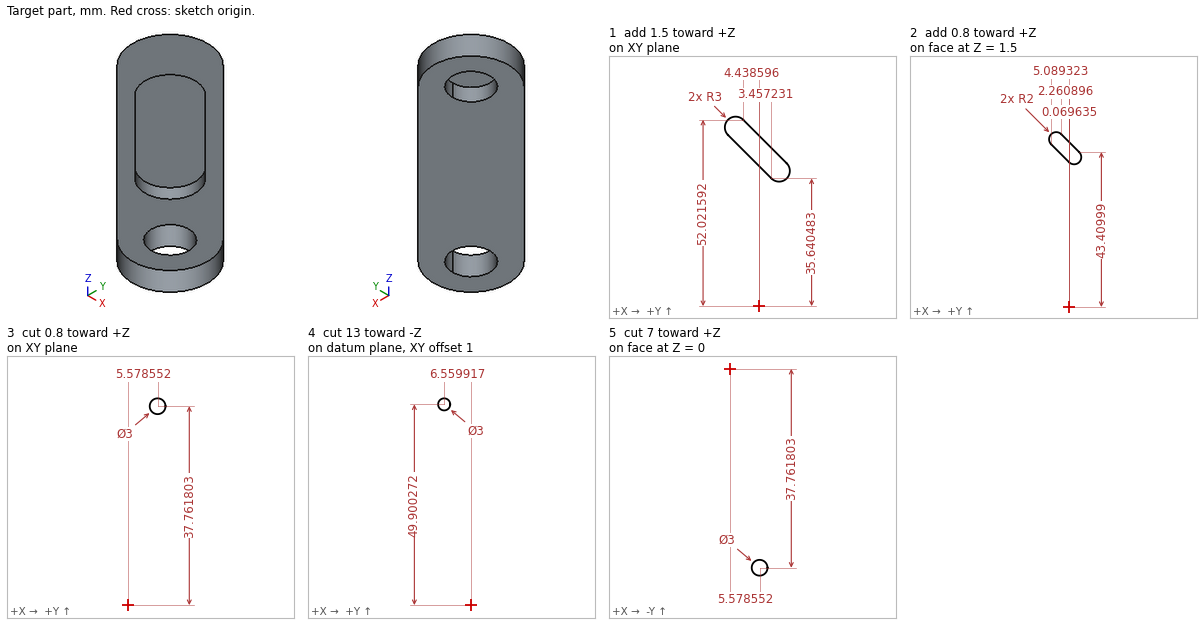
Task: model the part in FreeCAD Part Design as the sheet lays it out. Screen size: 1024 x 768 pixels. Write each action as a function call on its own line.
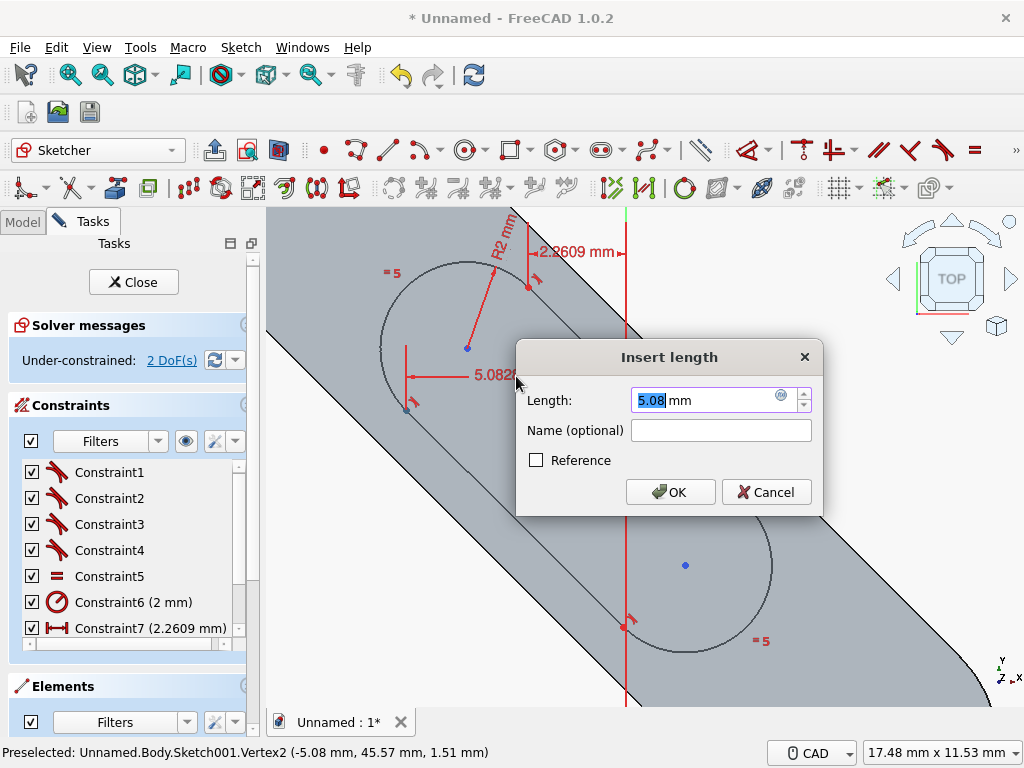
text(5.089323)
key(Return)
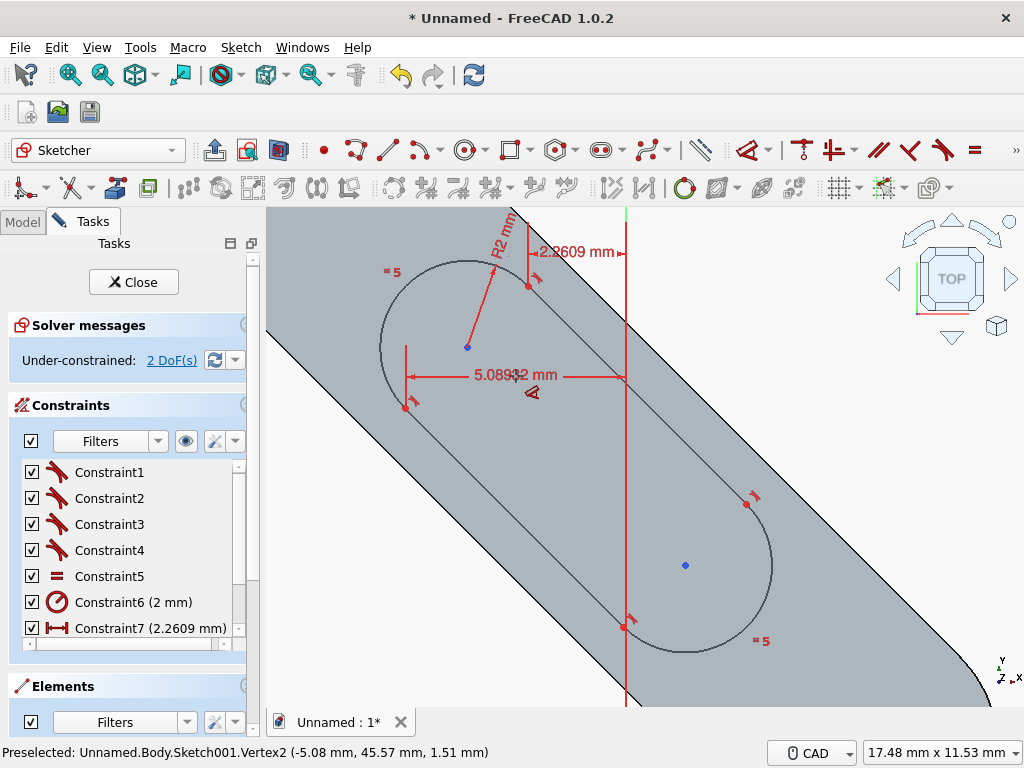
scroll(624, 627, up, 13)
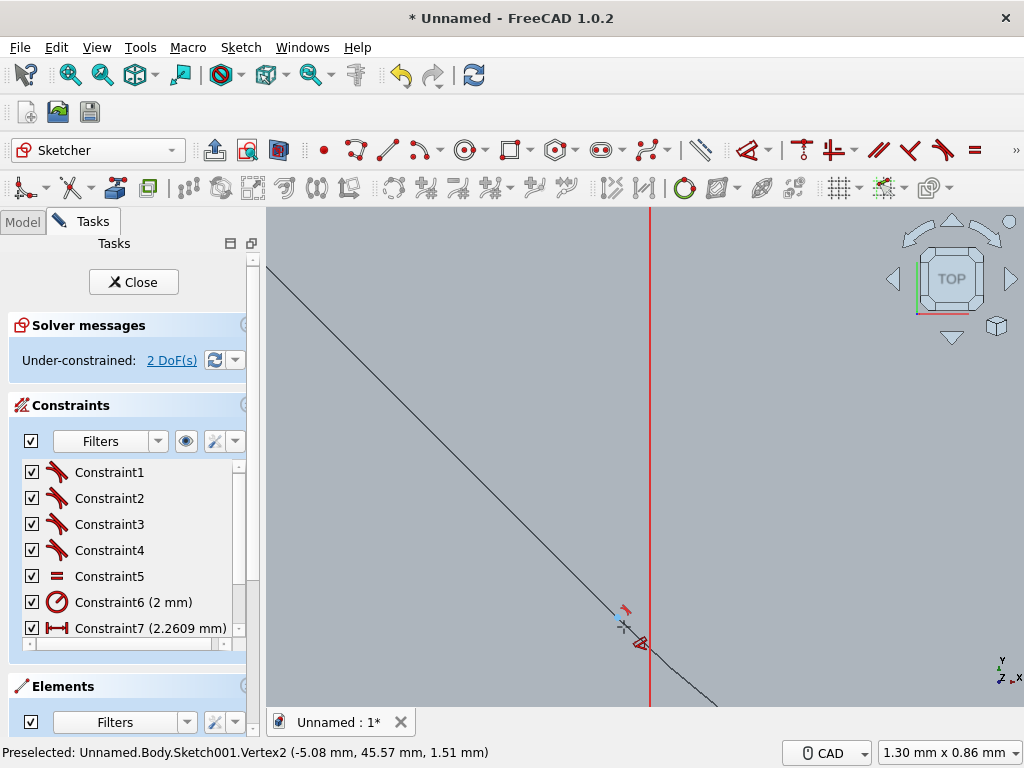
click(618, 618)
click(634, 584)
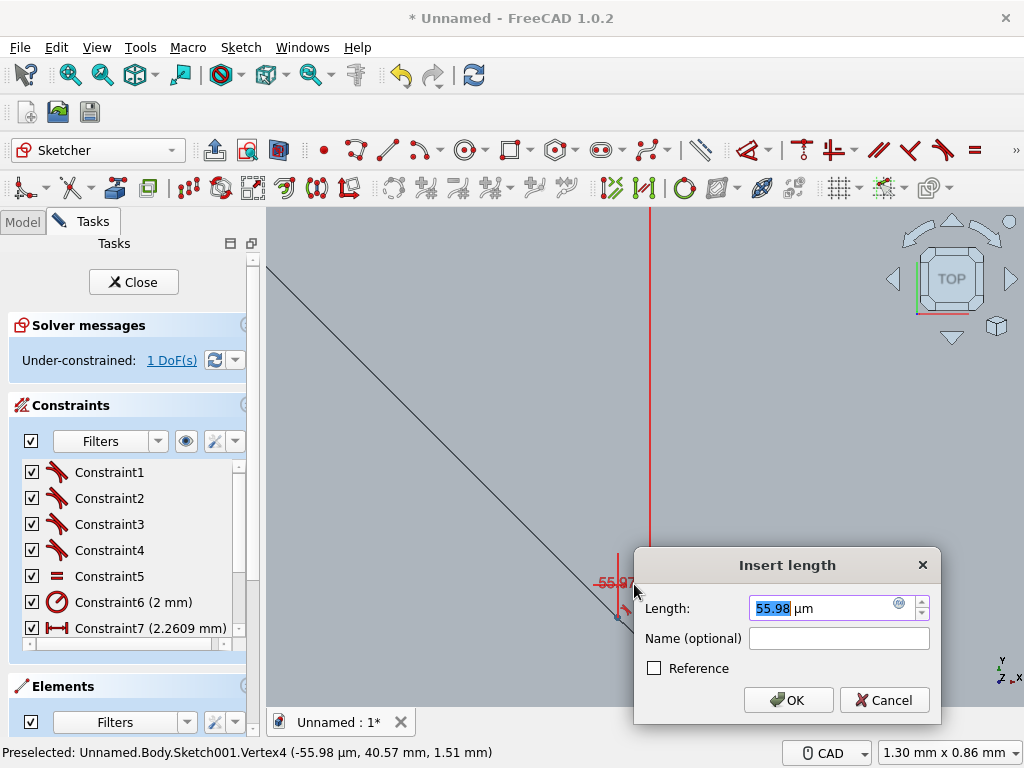
key(ctrl+a)
text(0.069635 mm)
key(Return)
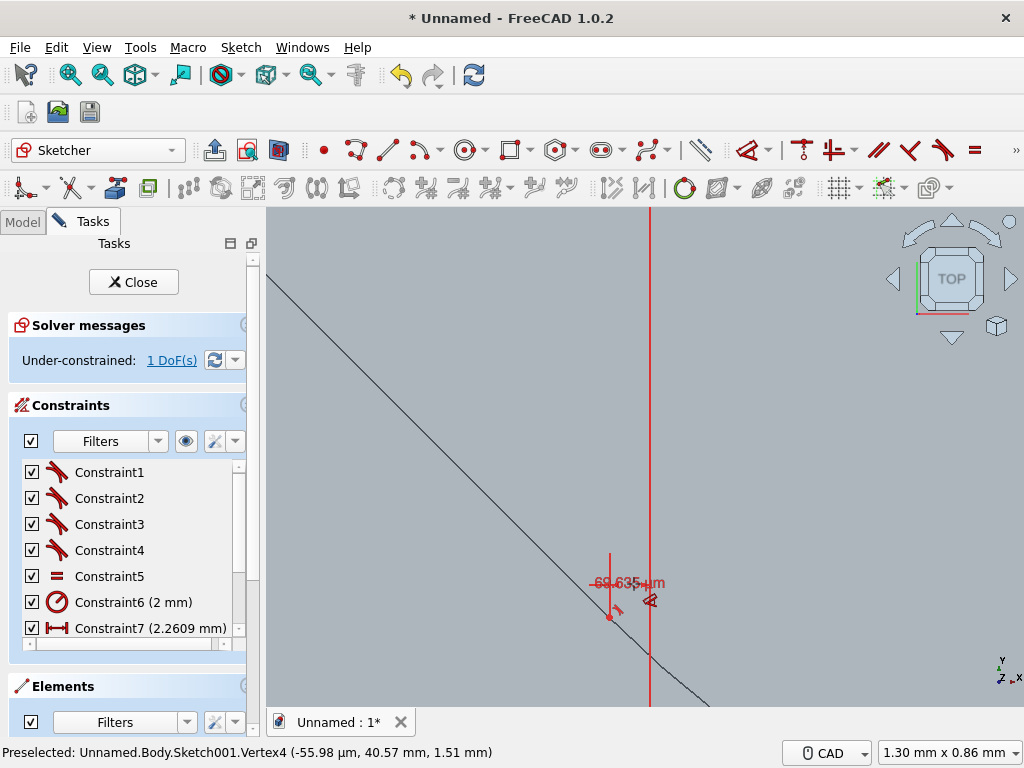
scroll(625, 628, down, 13)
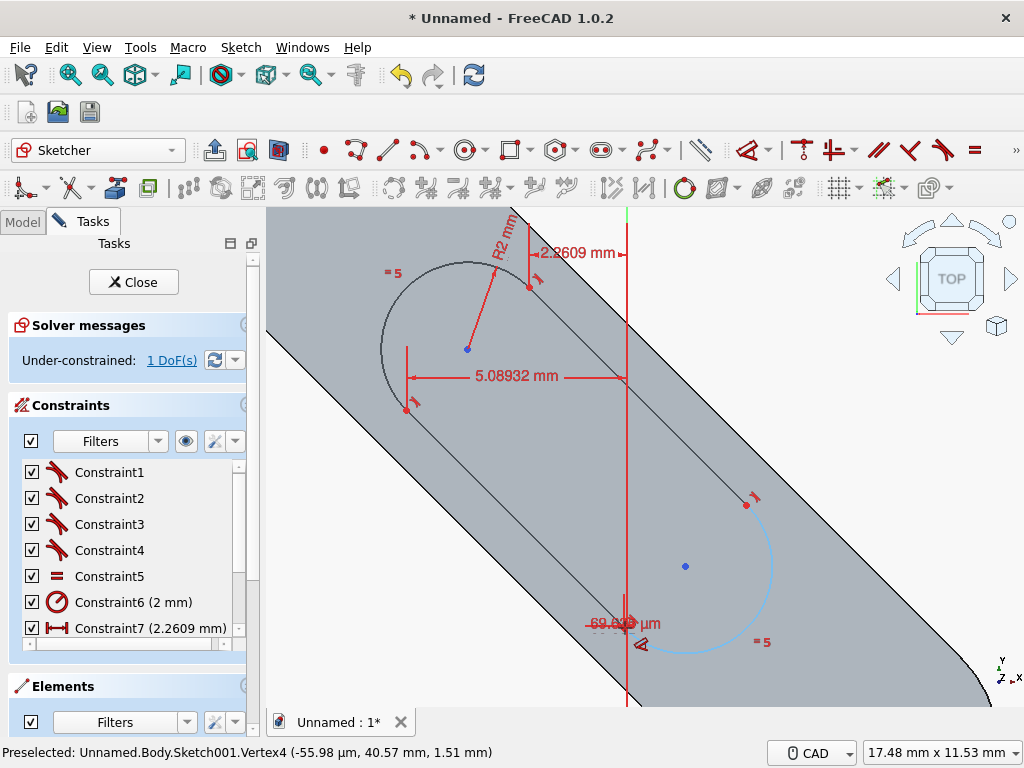
click(747, 505)
click(781, 632)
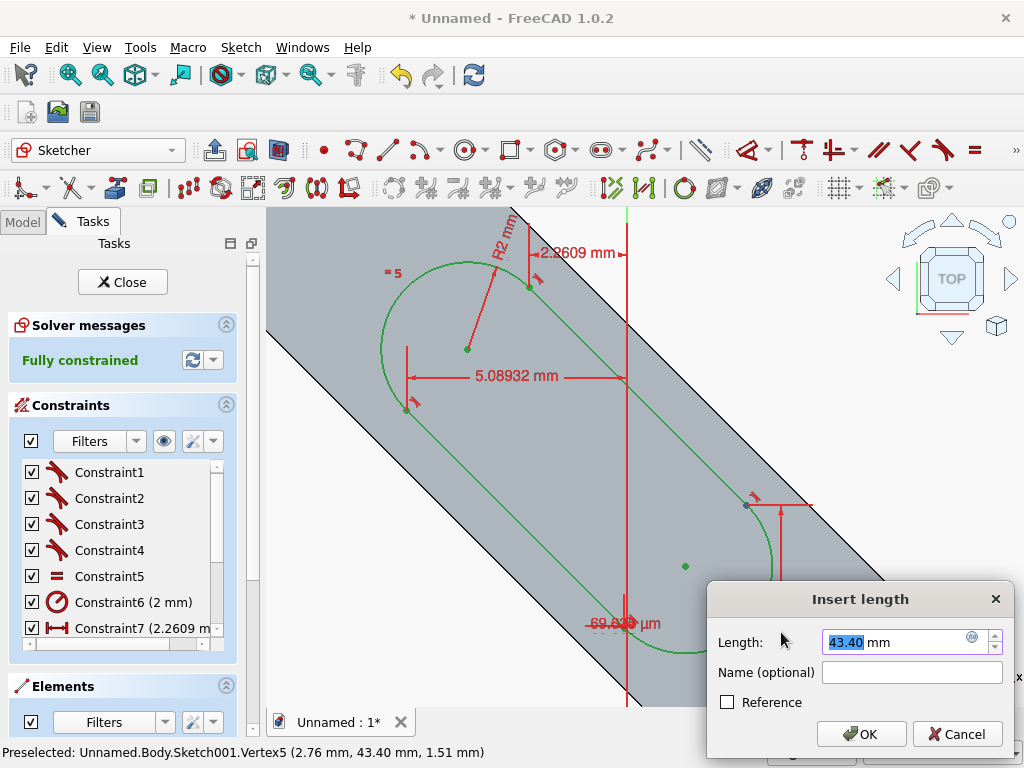
text(43.40999)
key(Return)
key(Escape)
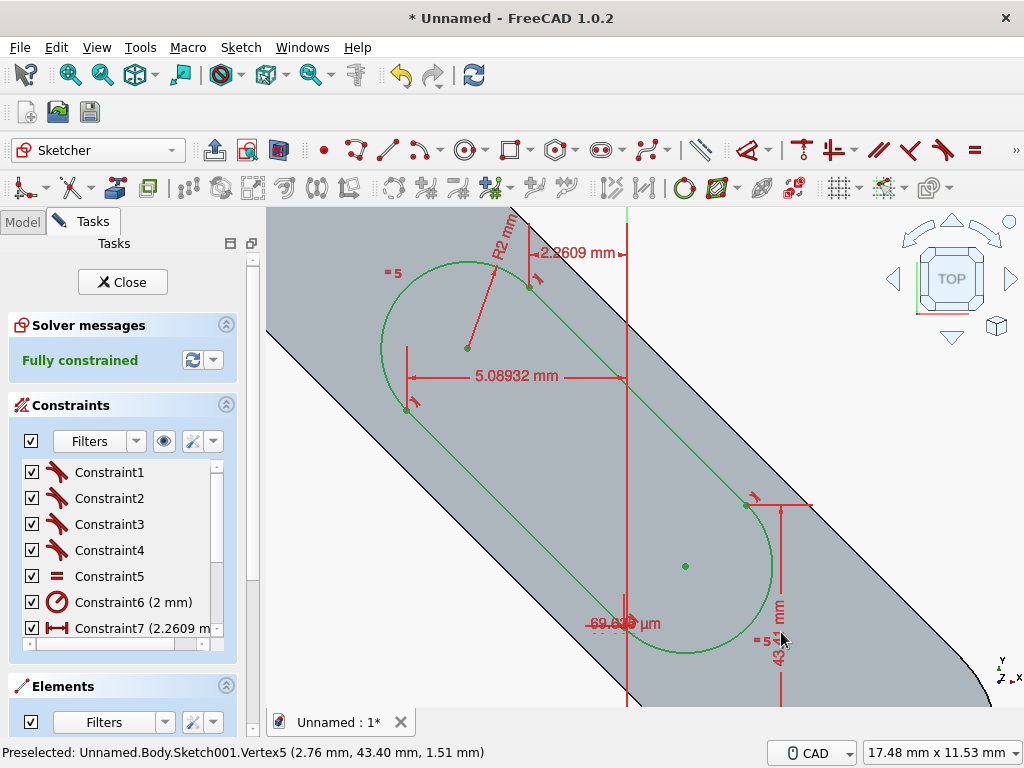
click(123, 282)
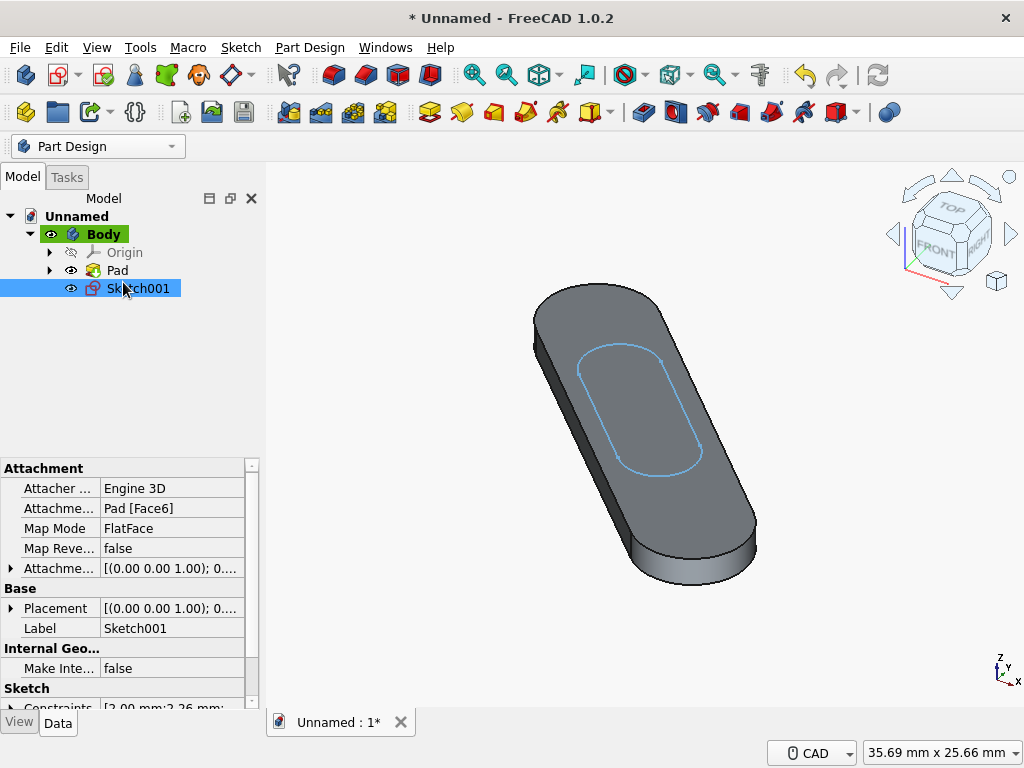
click(430, 112)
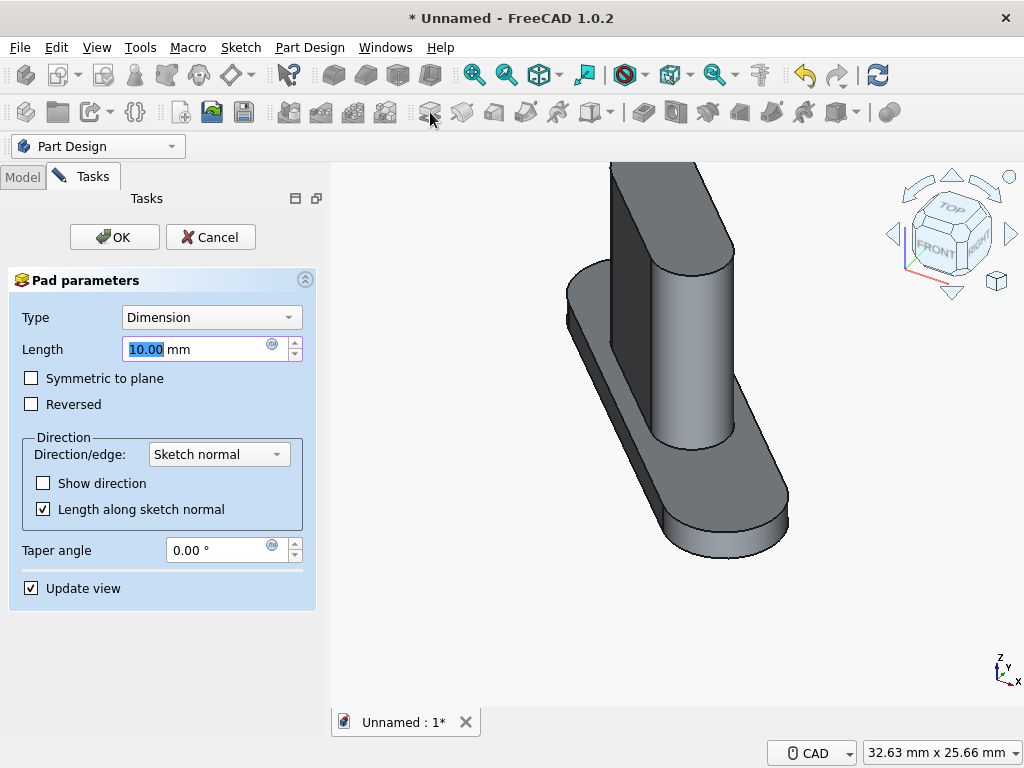
text(0.8)
key(Tab)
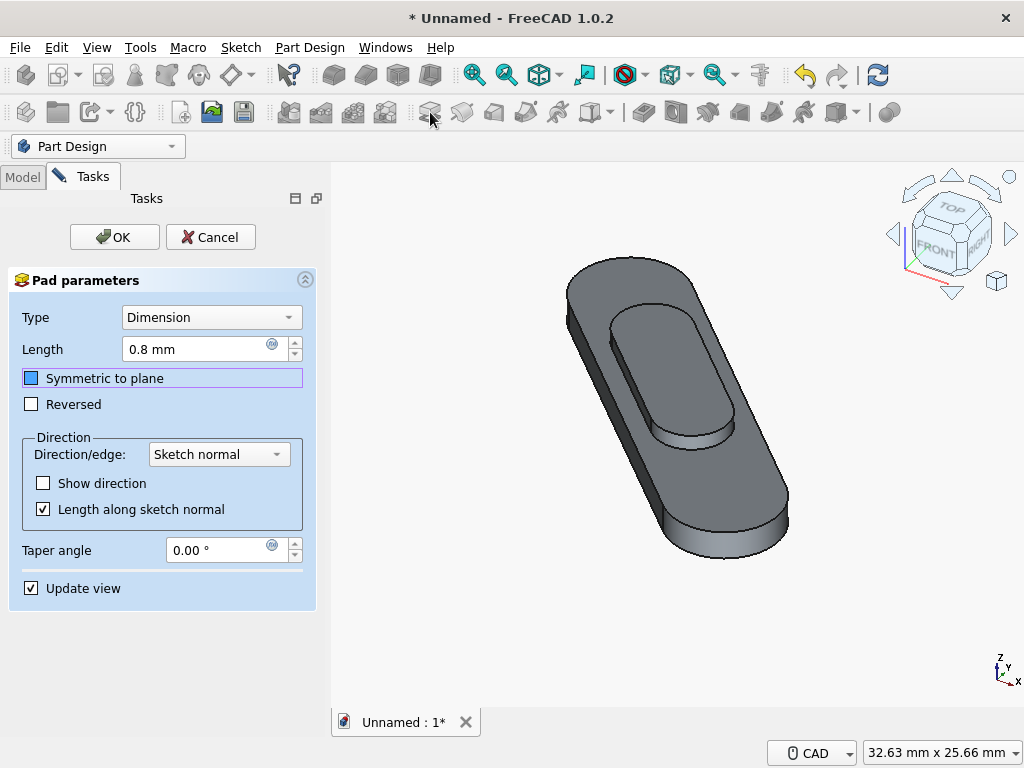
click(115, 237)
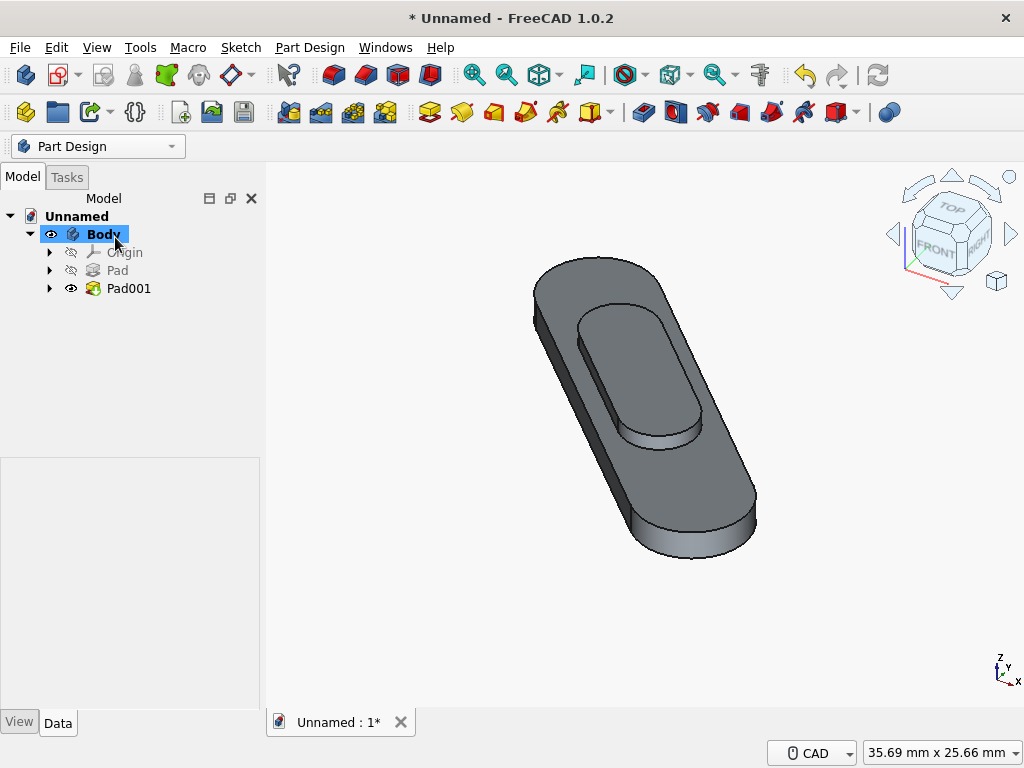
click(58, 76)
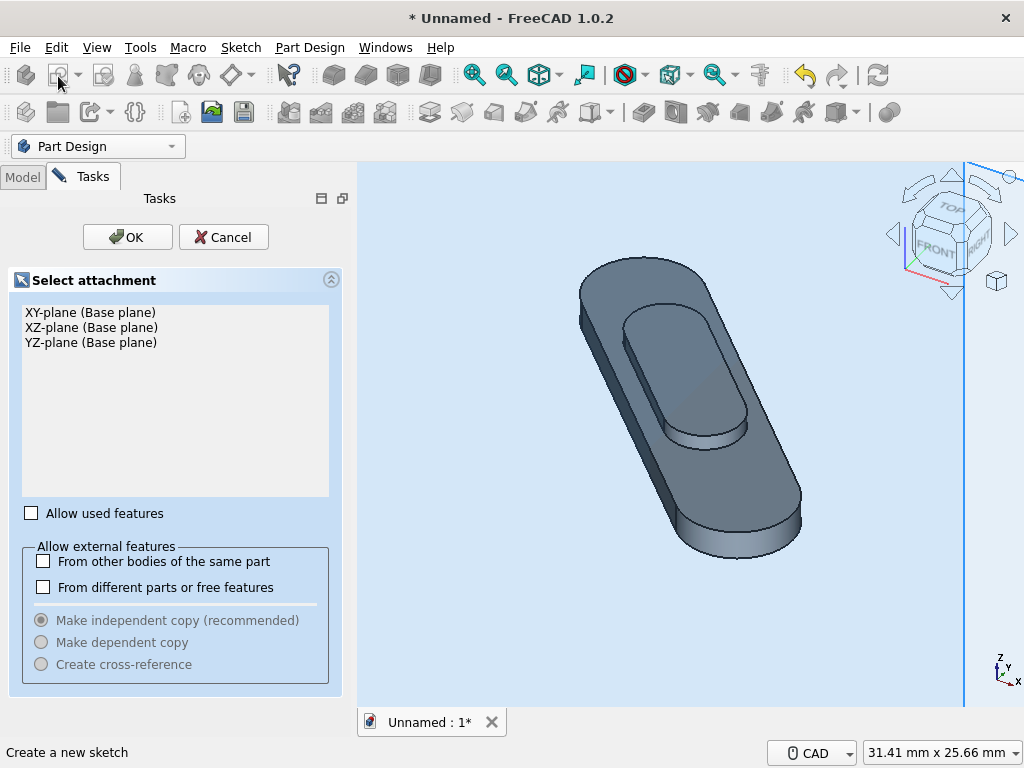
click(82, 312)